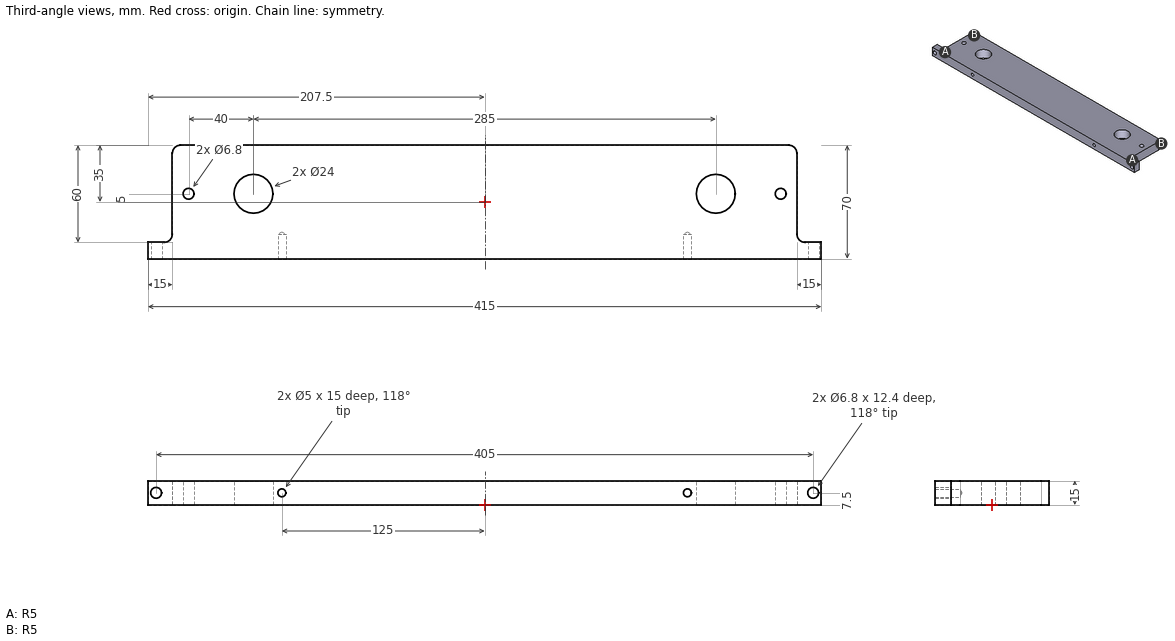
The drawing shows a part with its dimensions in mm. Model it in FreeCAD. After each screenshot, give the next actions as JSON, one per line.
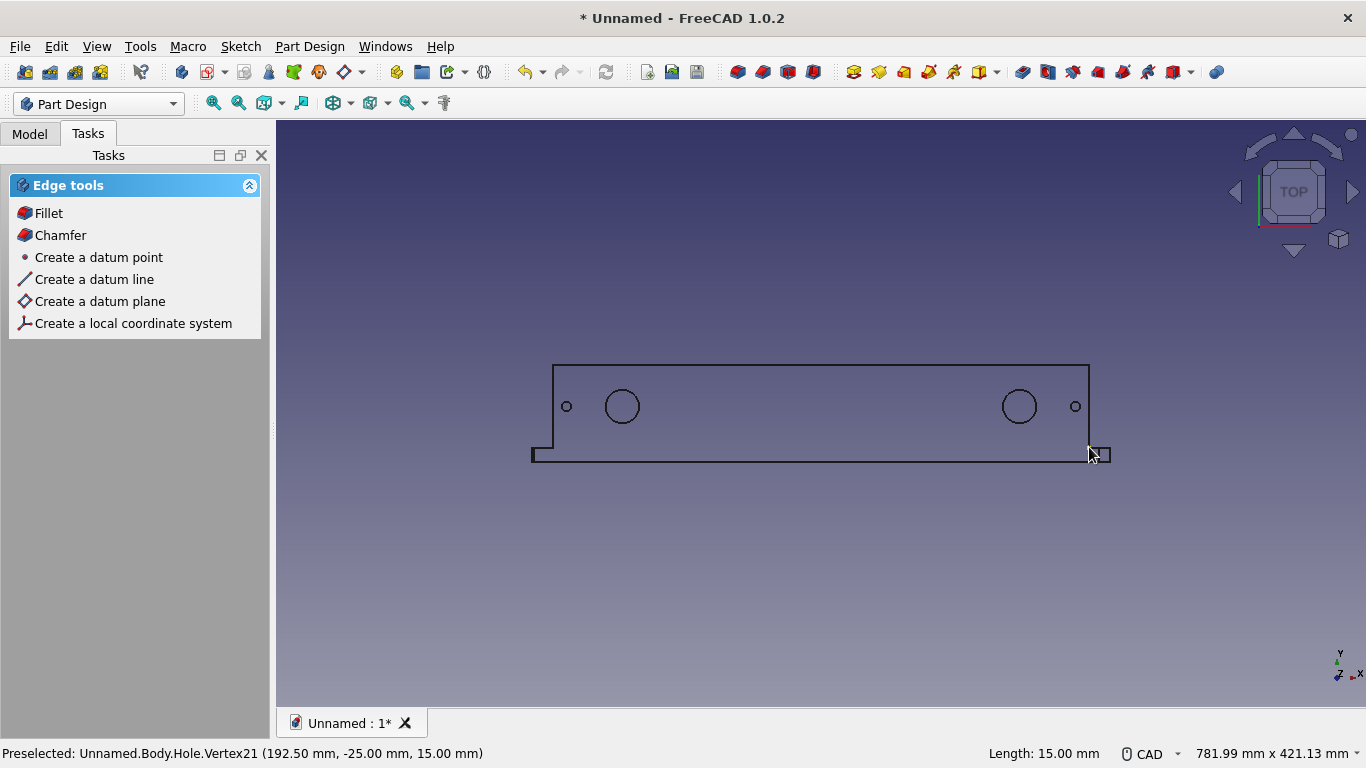
{"action": "key", "text": "1"}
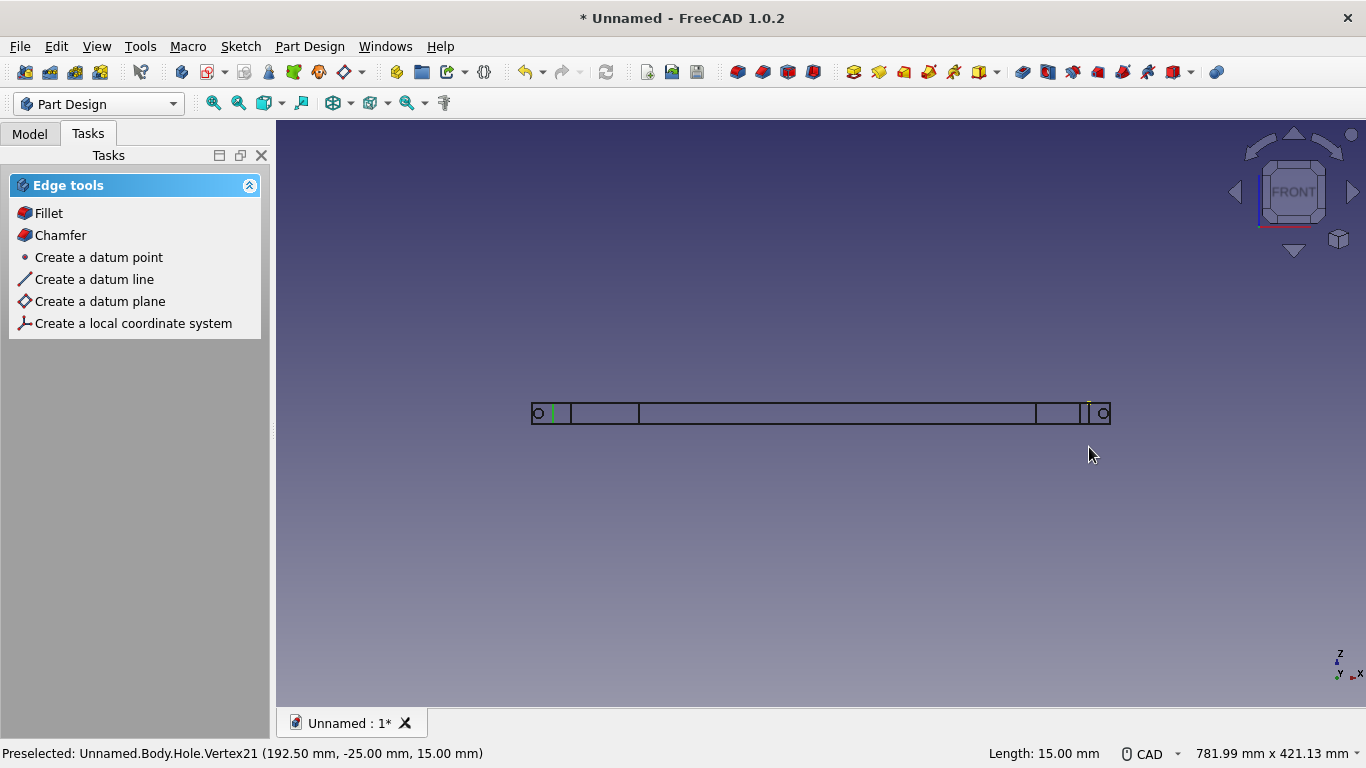
{"action": "left_click", "coordinate": [1089, 412], "text": "ctrl"}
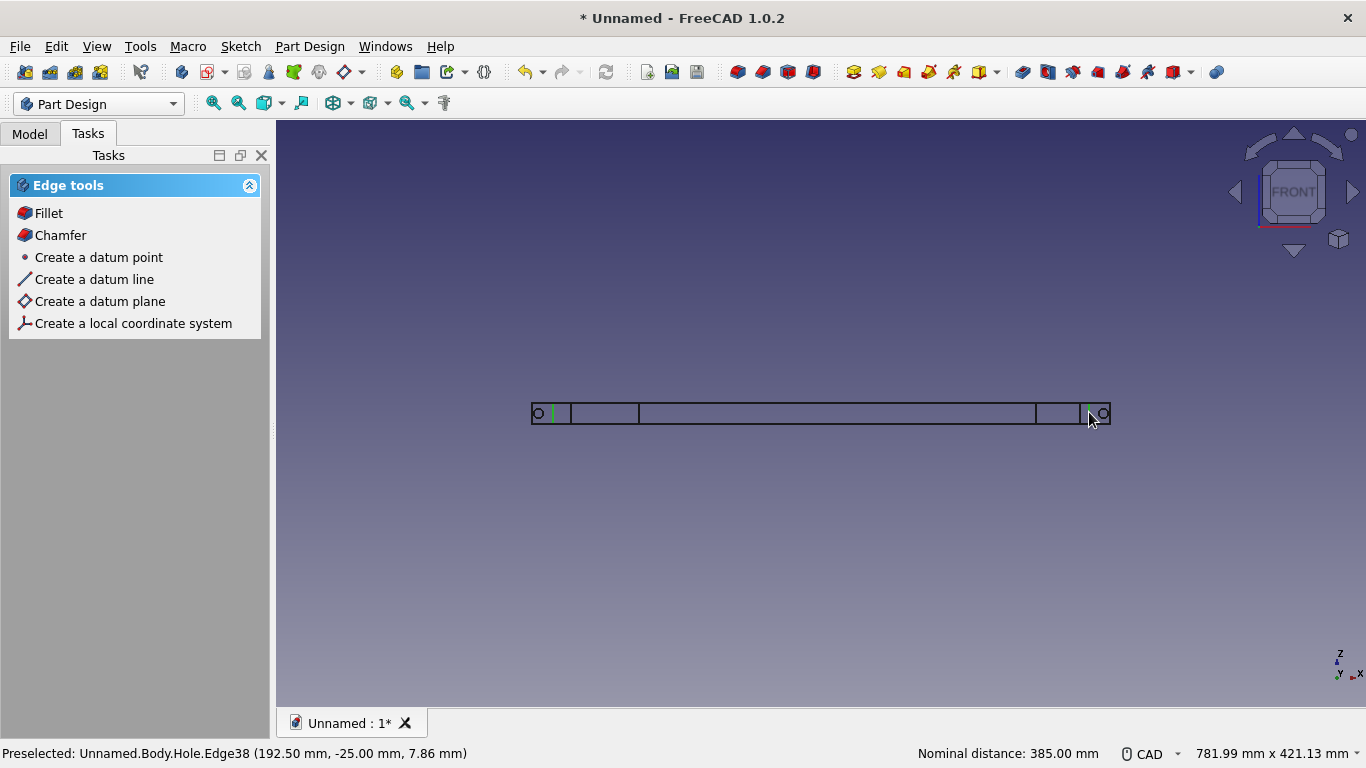
{"action": "key", "text": "v 1"}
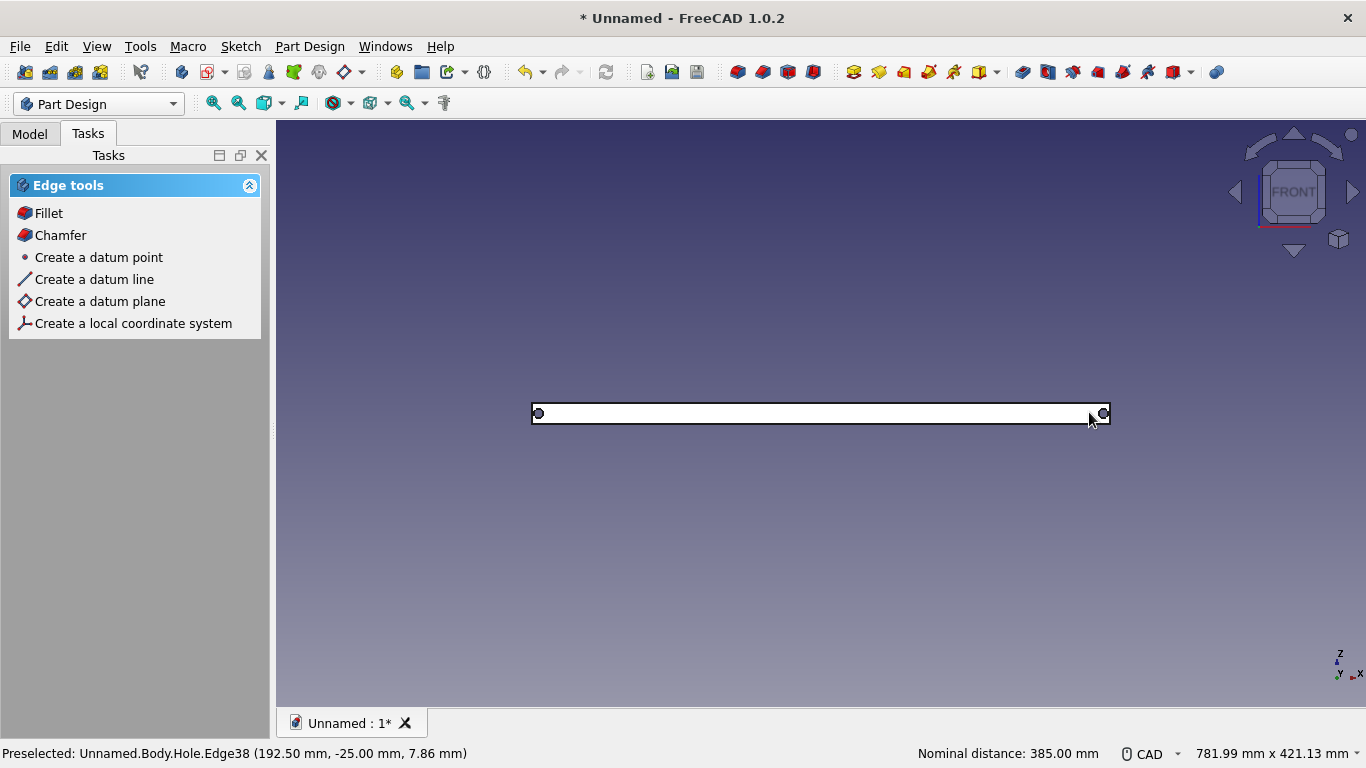
{"action": "left_click", "coordinate": [738, 72]}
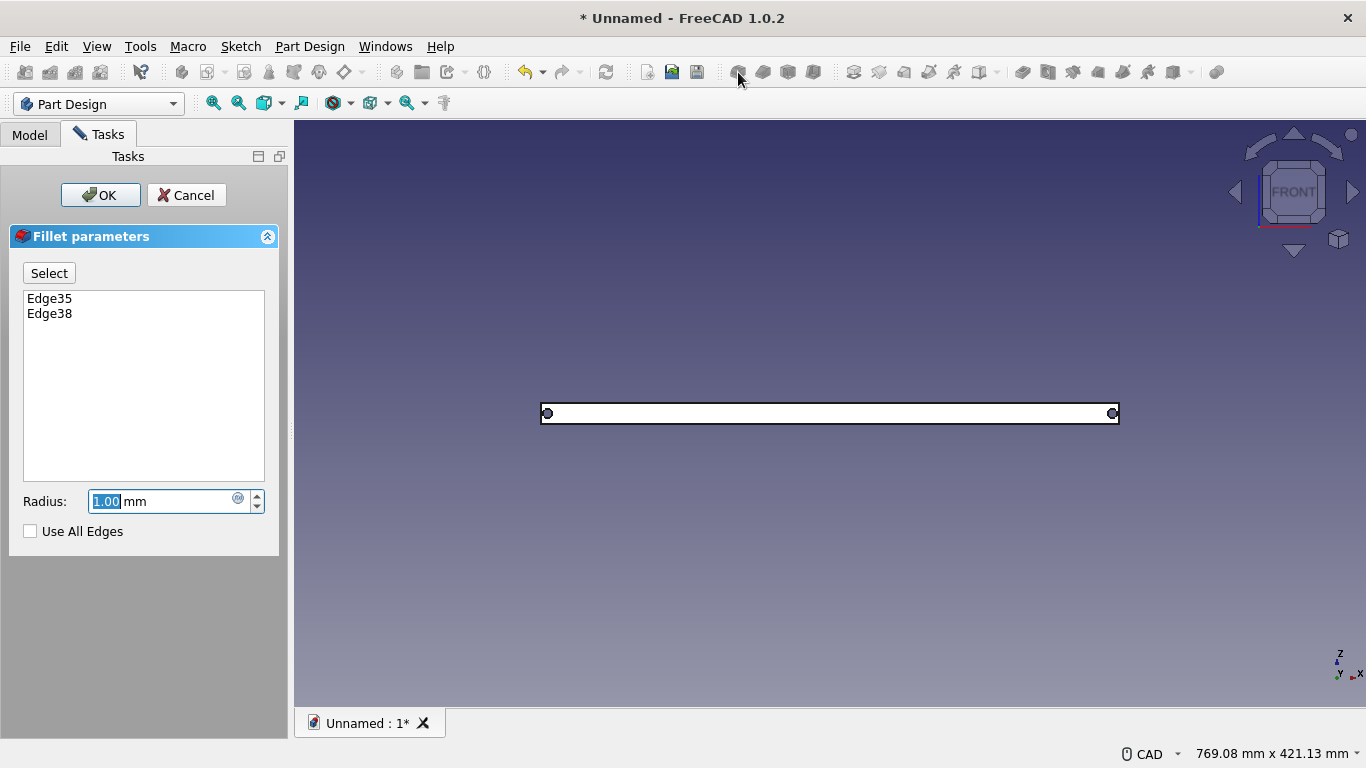
{"action": "type", "text": "5"}
{"action": "key", "text": "Tab"}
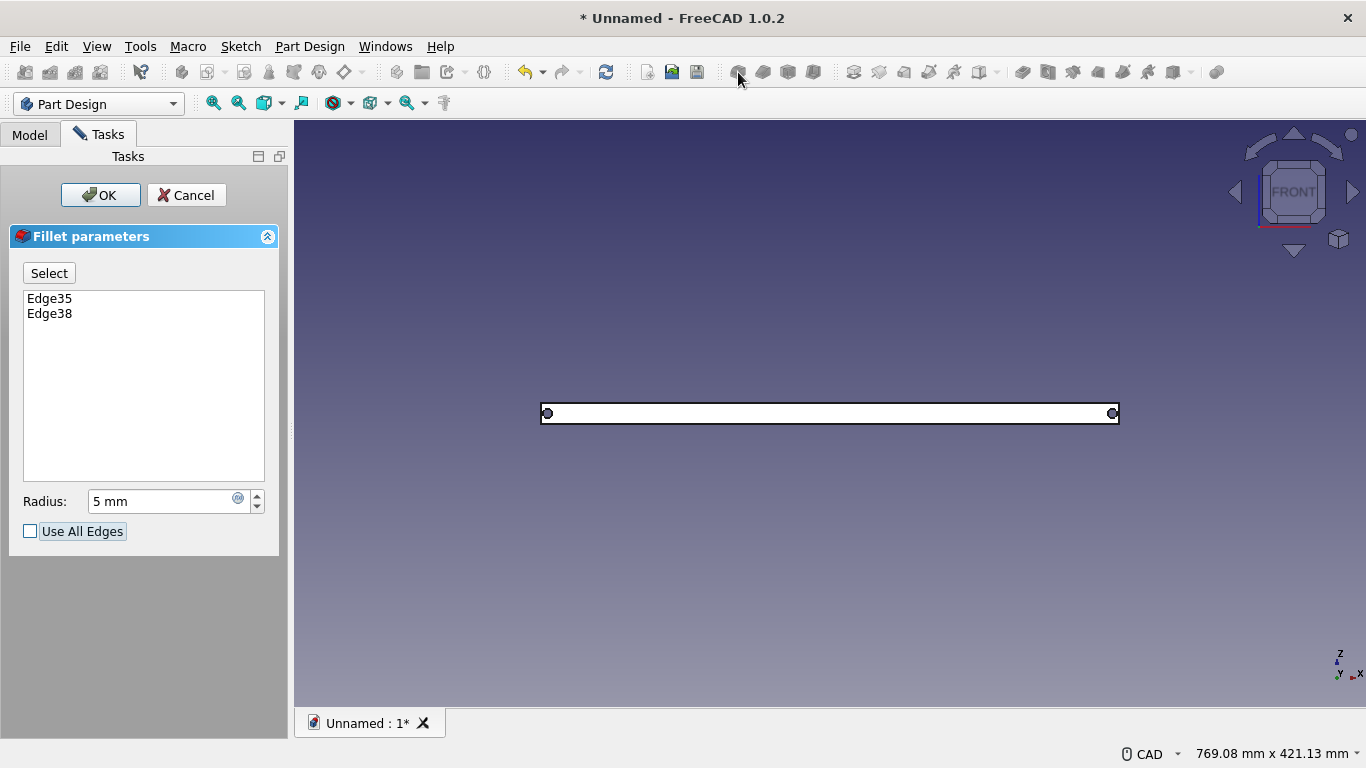
{"action": "left_click", "coordinate": [101, 195]}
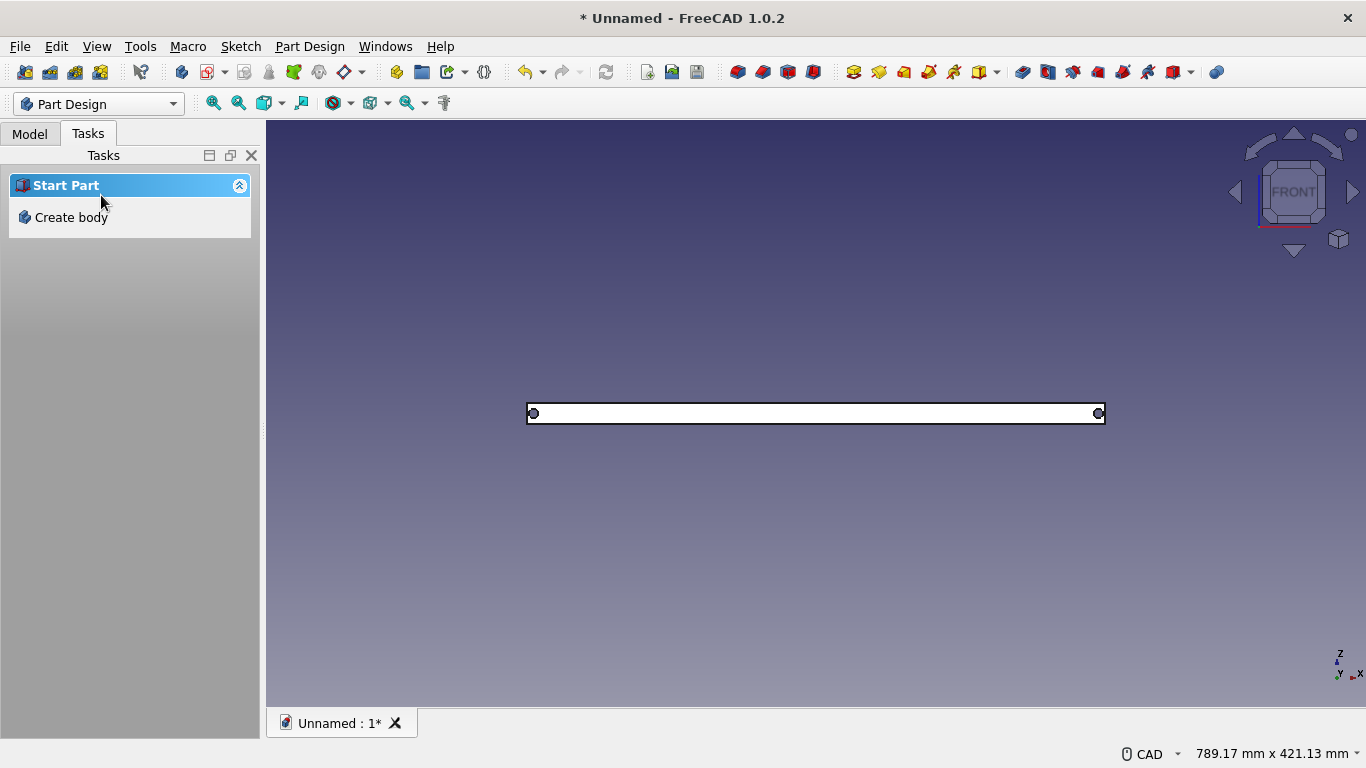
{"action": "scroll", "coordinate": [548, 412], "scroll_direction": "up", "scroll_amount": 4}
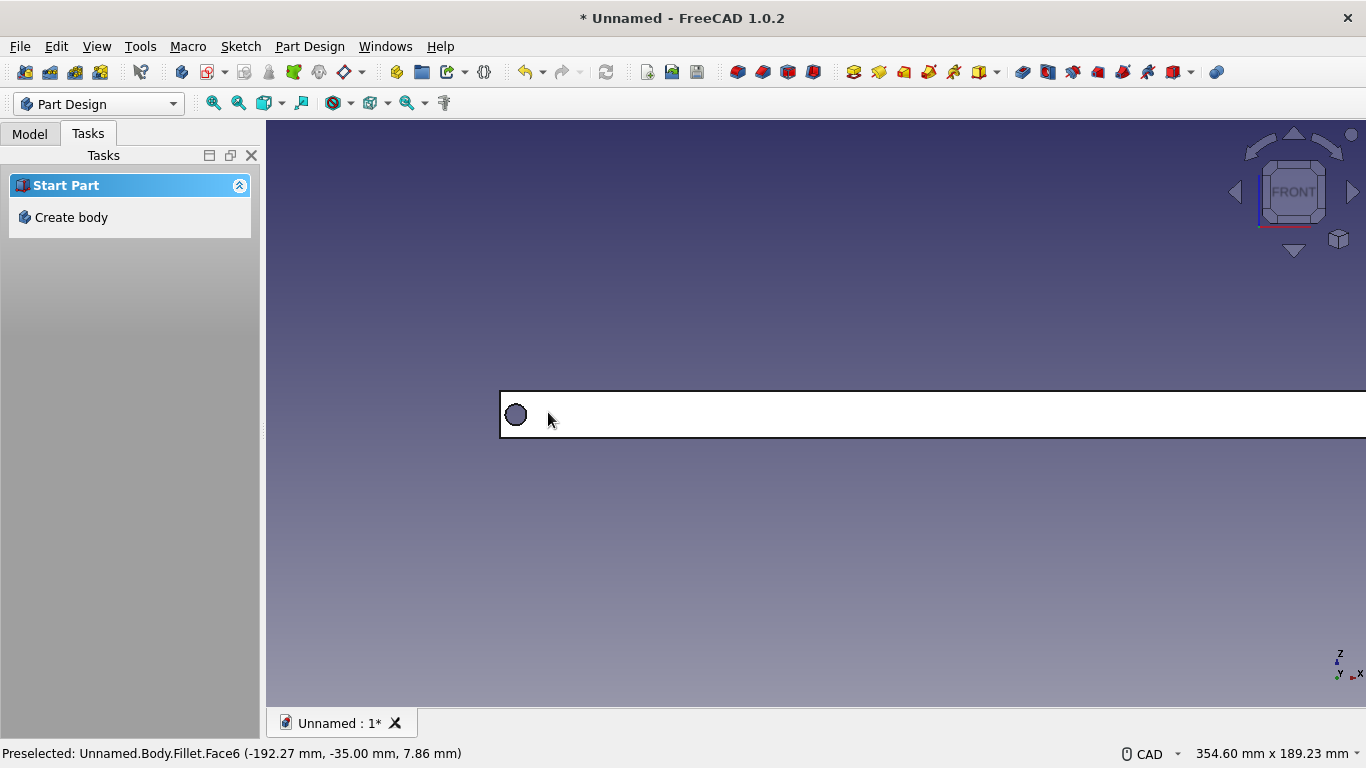
{"action": "key", "text": "v f"}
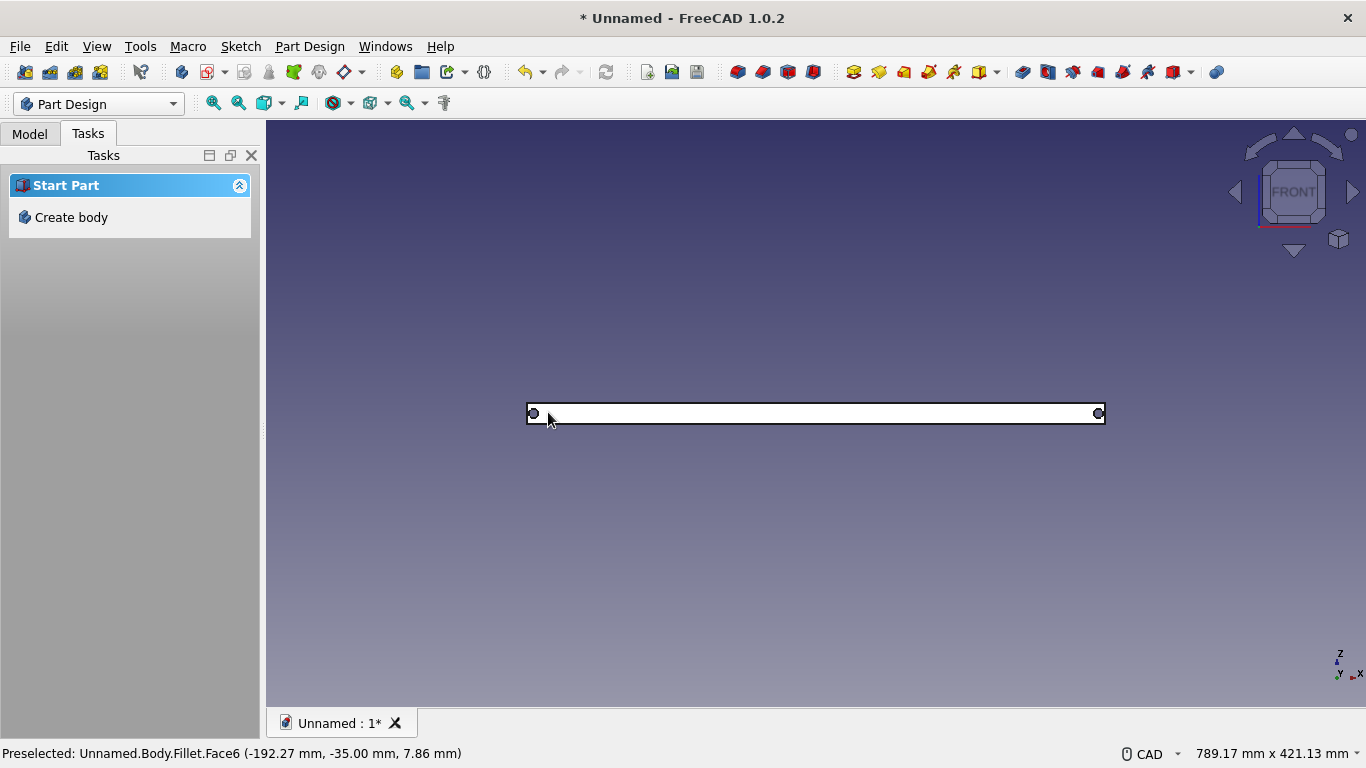
{"action": "key", "text": "0"}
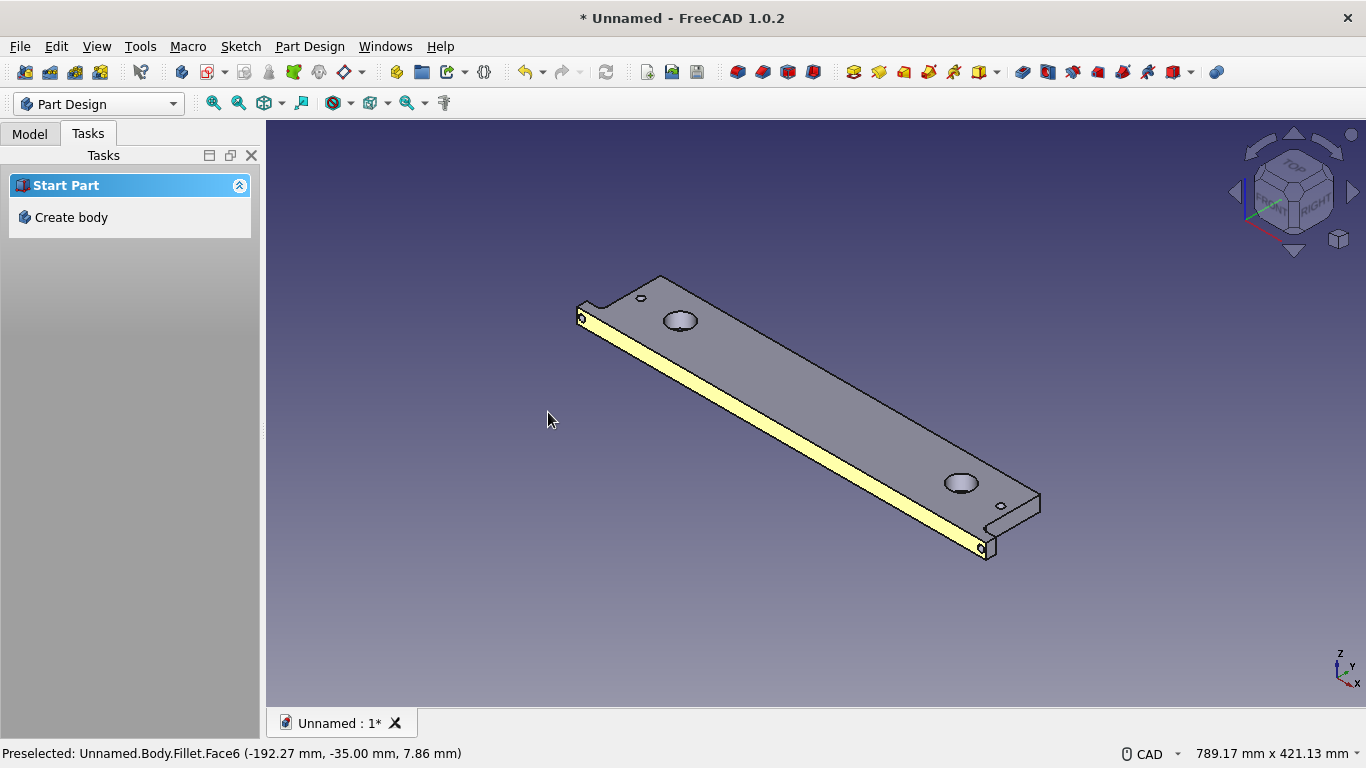
{"action": "scroll", "coordinate": [661, 283], "scroll_direction": "up", "scroll_amount": 4}